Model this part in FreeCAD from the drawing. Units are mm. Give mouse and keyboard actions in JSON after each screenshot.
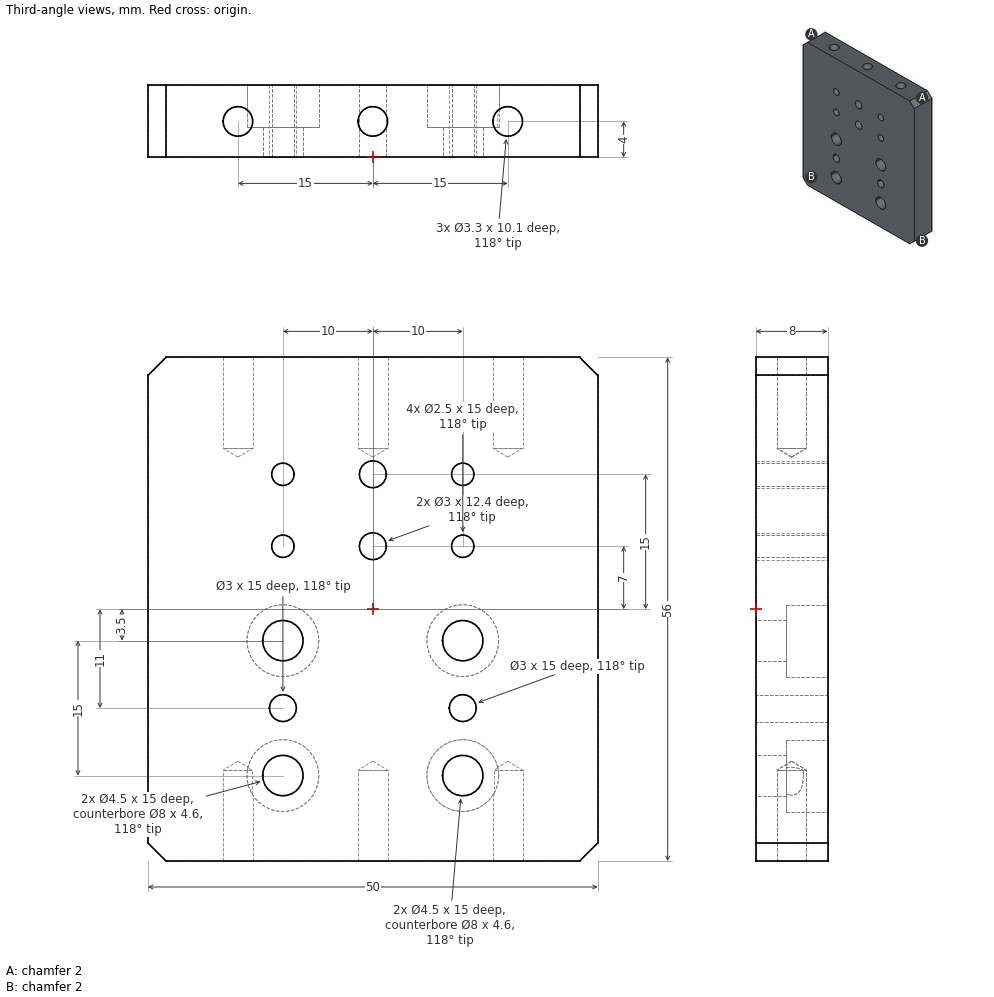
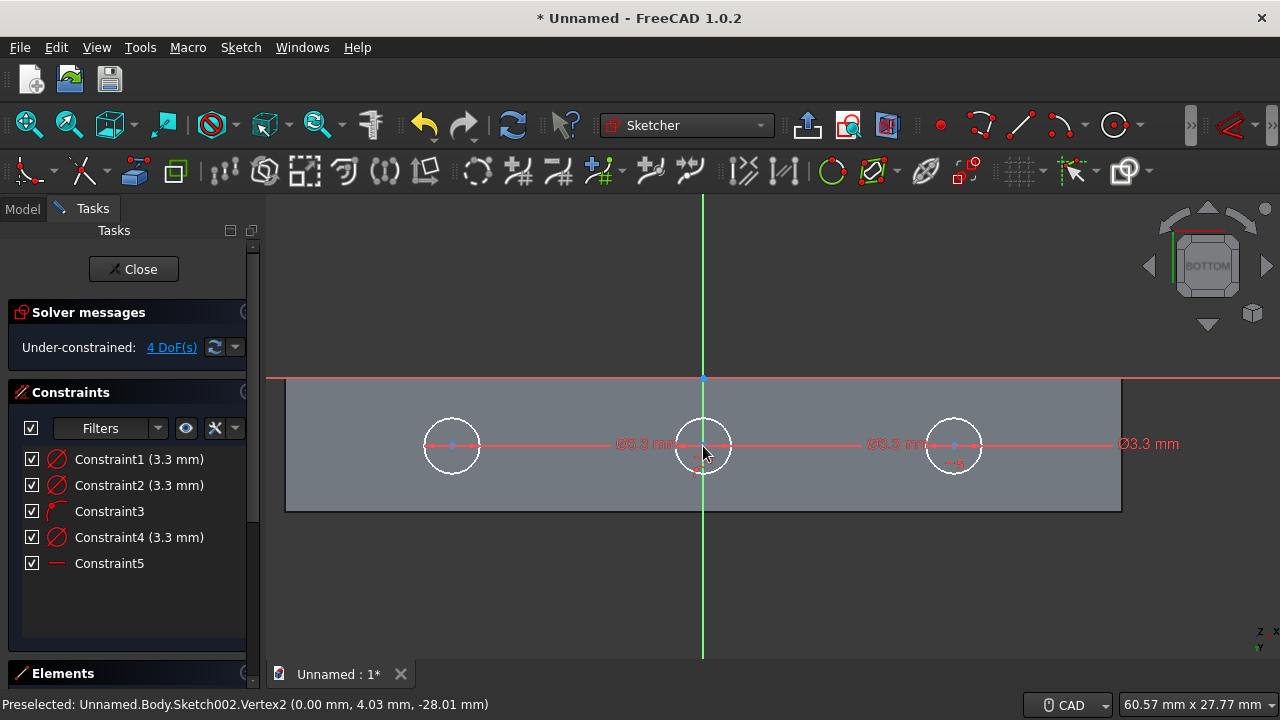
{"action": "left_click", "coordinate": [703, 446]}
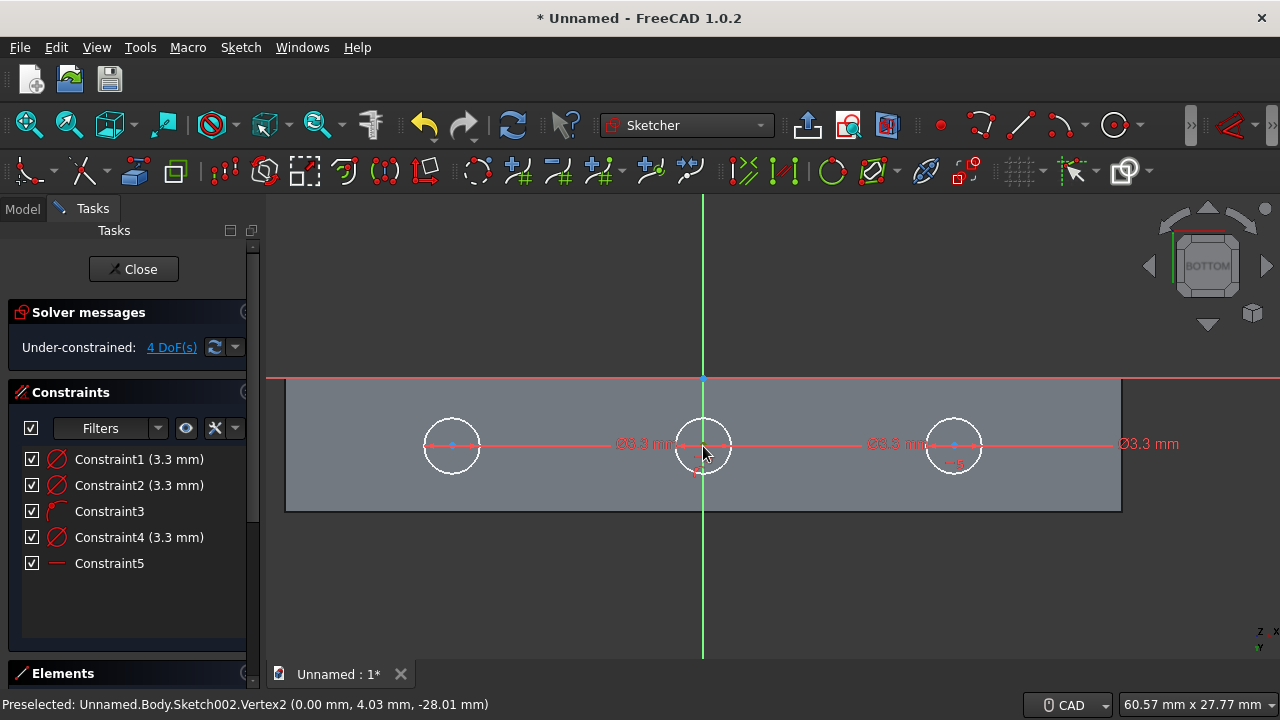
{"action": "left_click", "coordinate": [452, 446]}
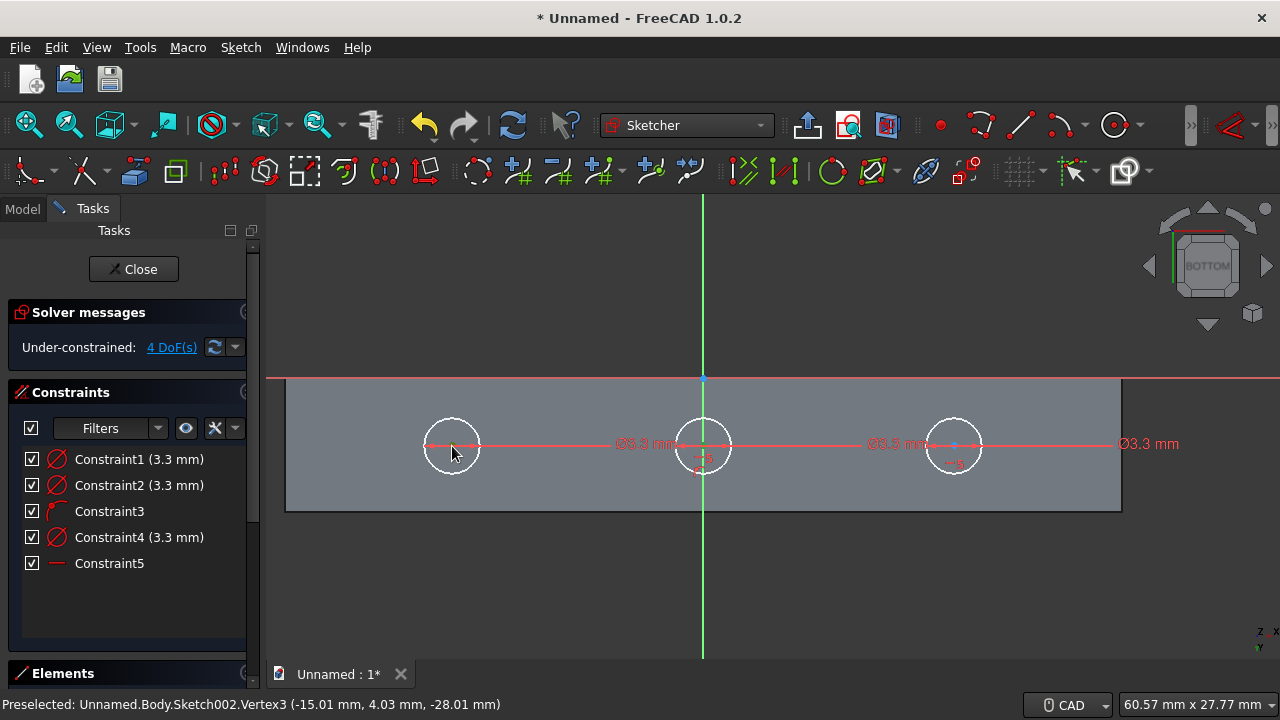
{"action": "key", "text": "h"}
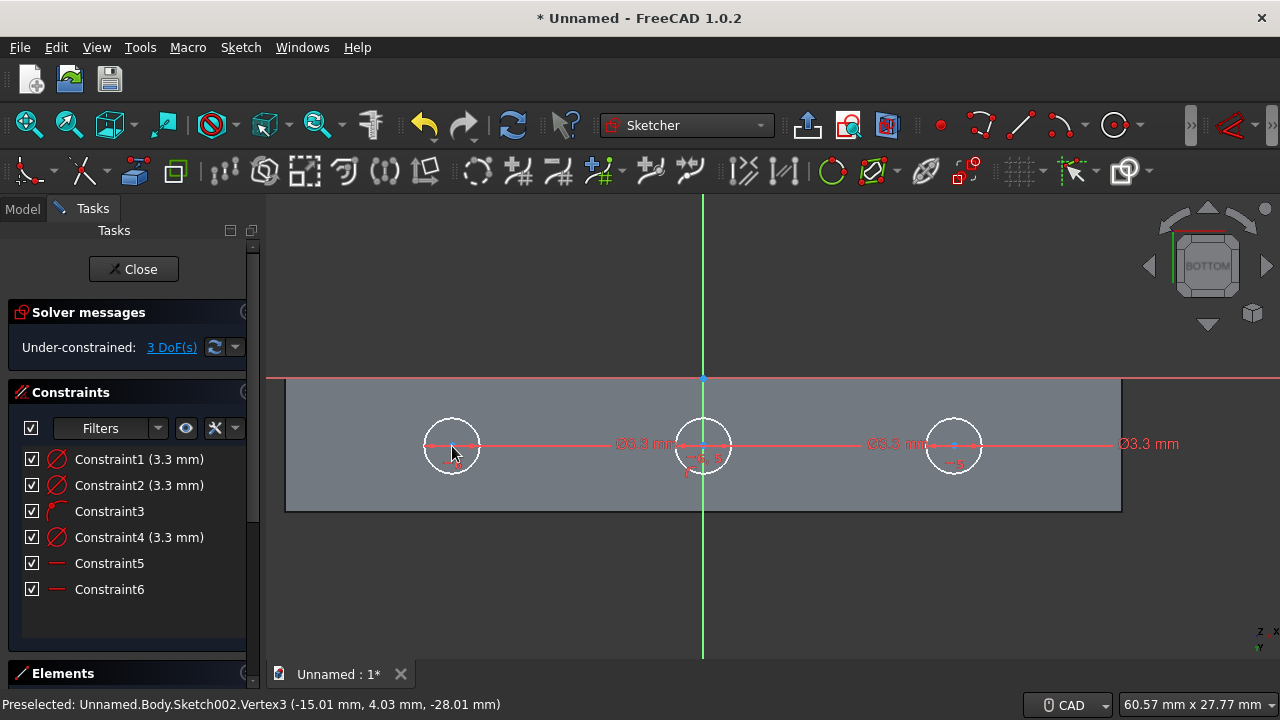
{"action": "left_click", "coordinate": [1230, 126]}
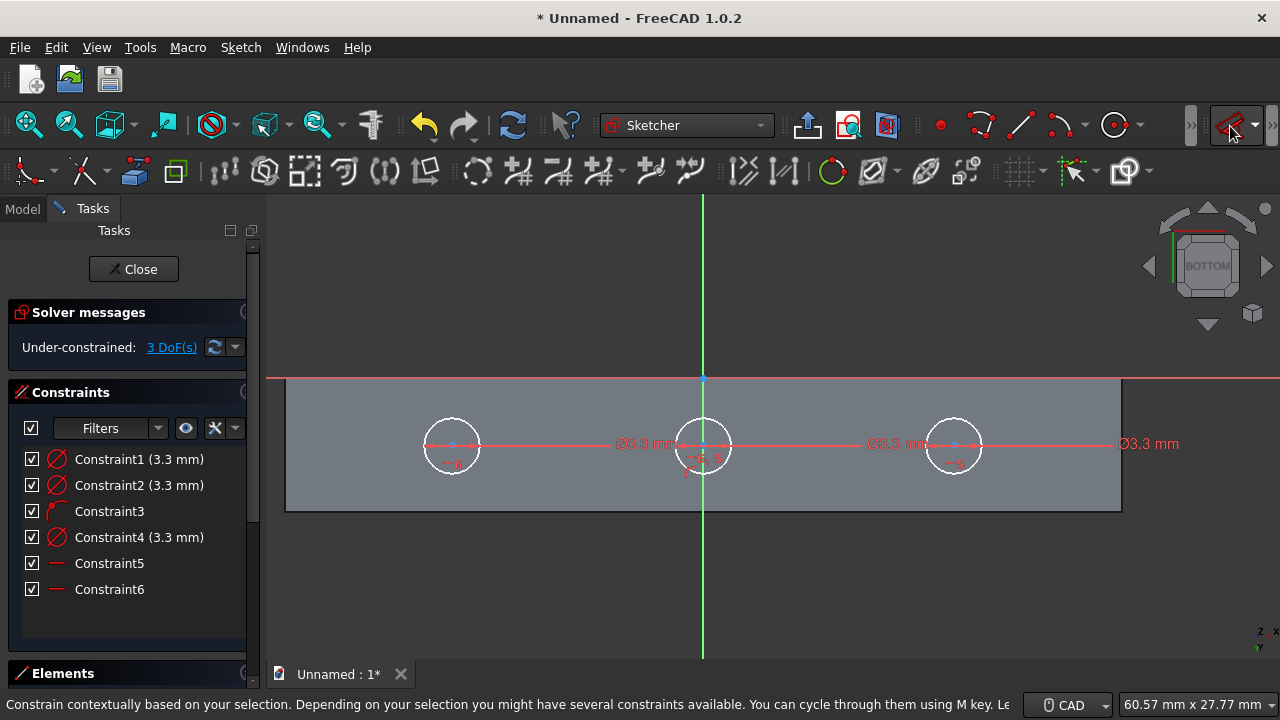
{"action": "left_click", "coordinate": [954, 446]}
{"action": "left_click", "coordinate": [988, 412]}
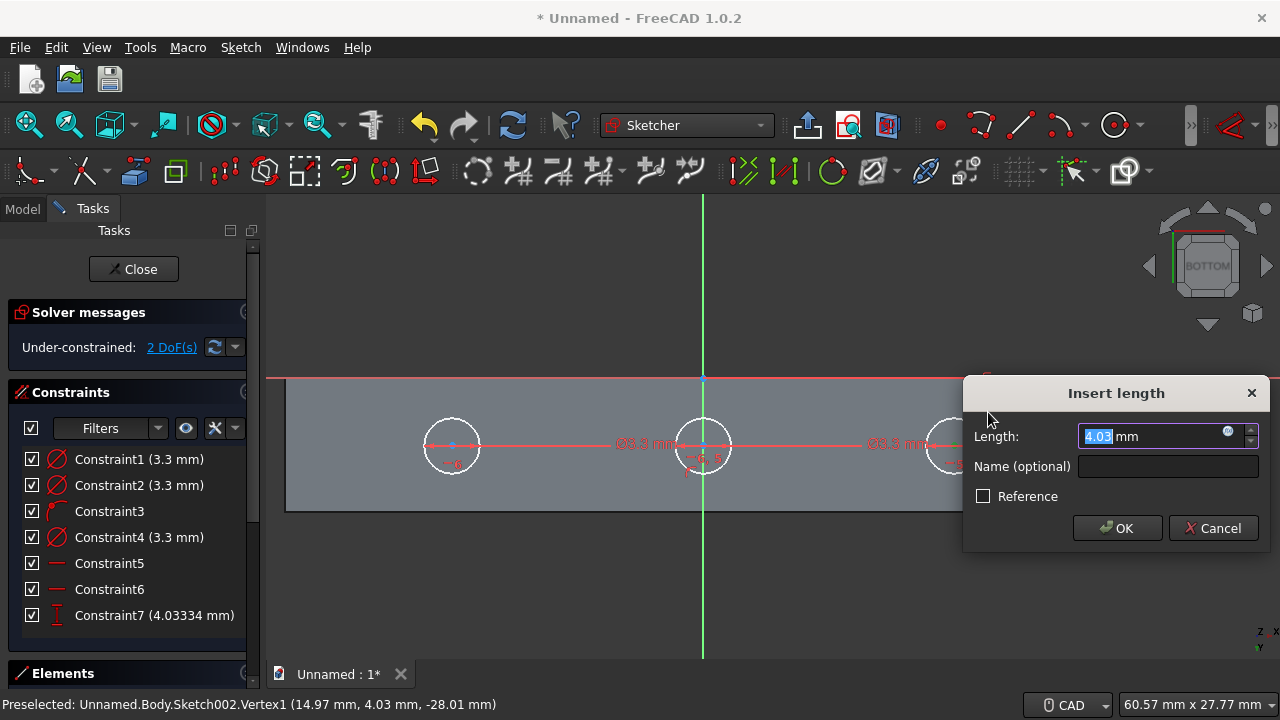
{"action": "type", "text": "4"}
{"action": "key", "text": "Return"}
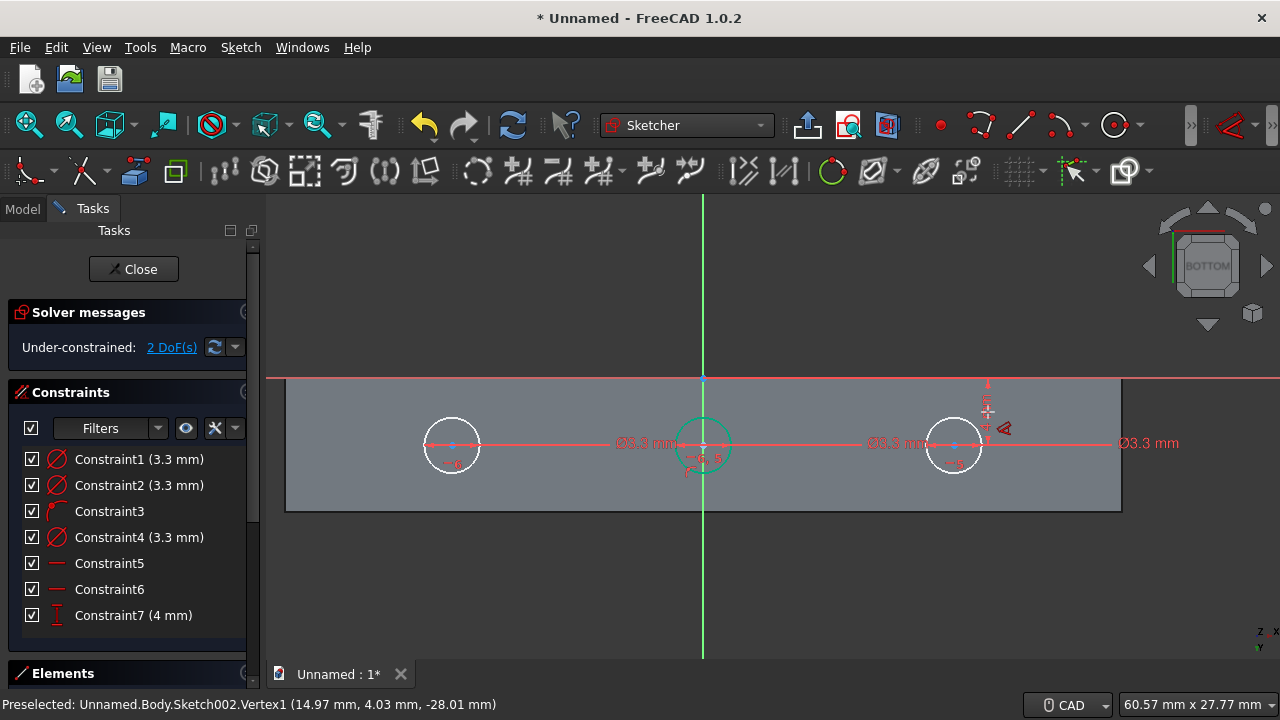
{"action": "left_click", "coordinate": [954, 445]}
{"action": "left_click", "coordinate": [829, 344]}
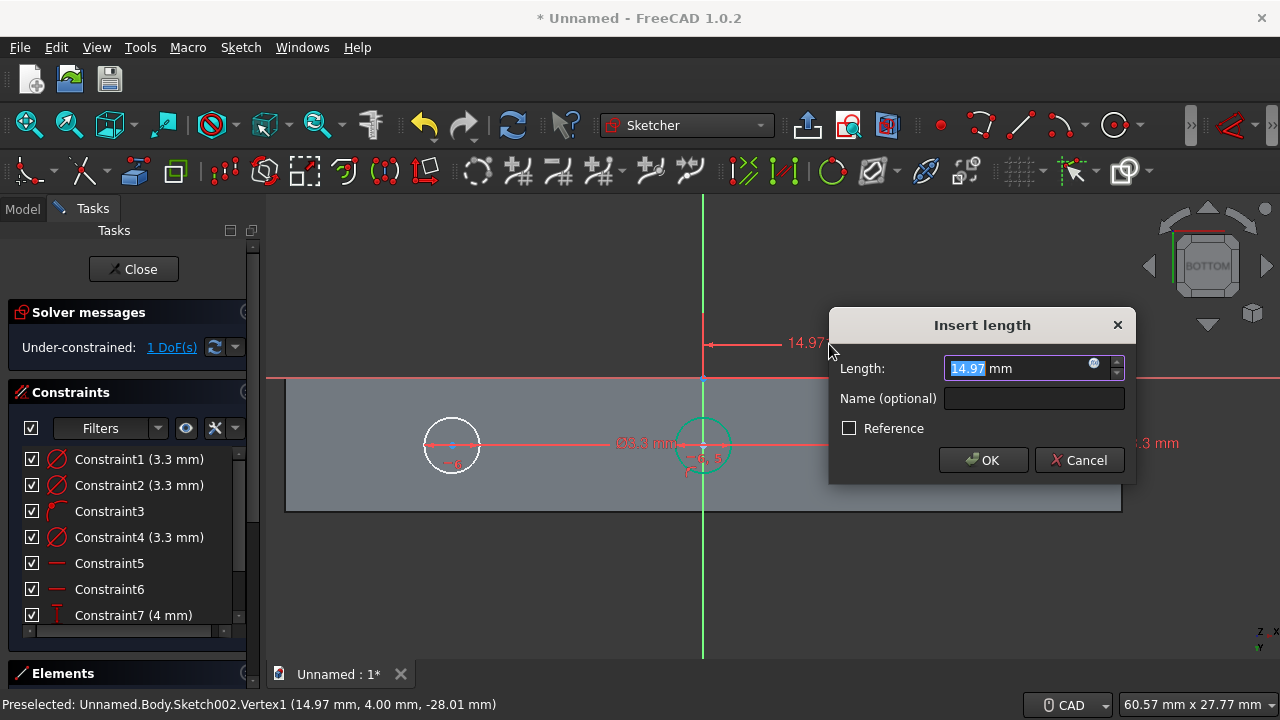
{"action": "type", "text": "15"}
{"action": "key", "text": "Return"}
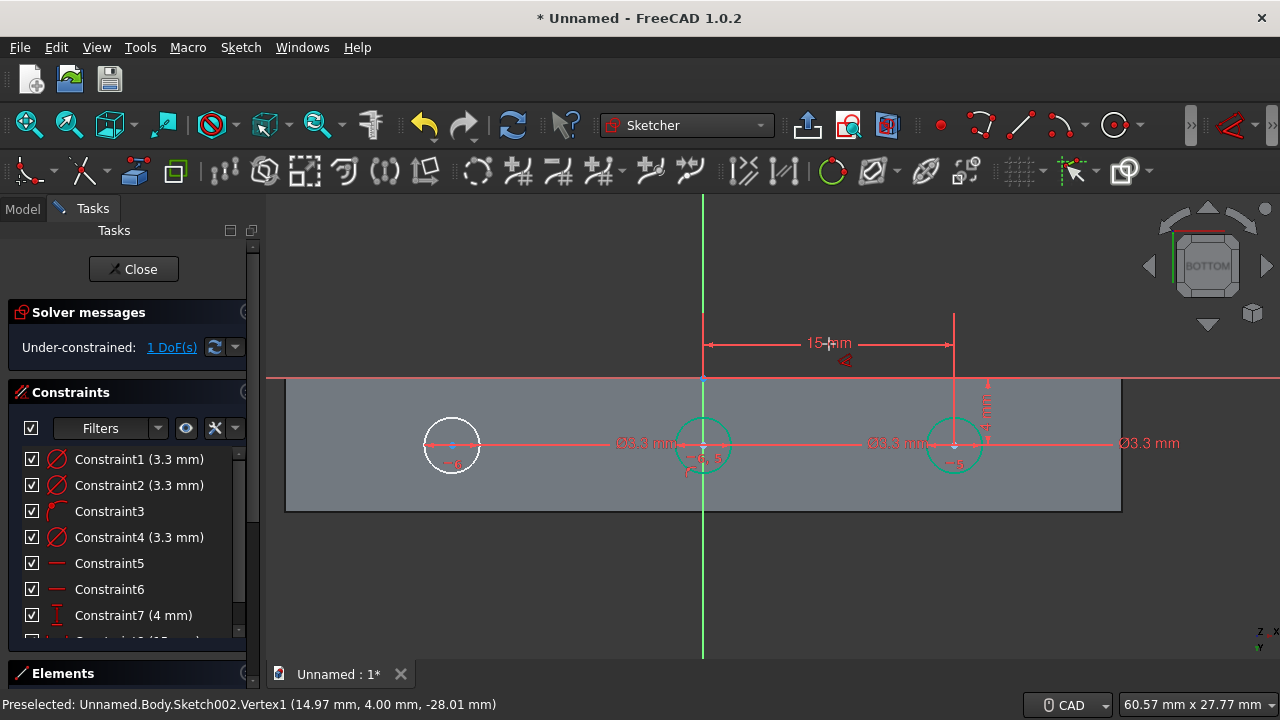
{"action": "left_click", "coordinate": [452, 445]}
{"action": "left_click", "coordinate": [578, 344]}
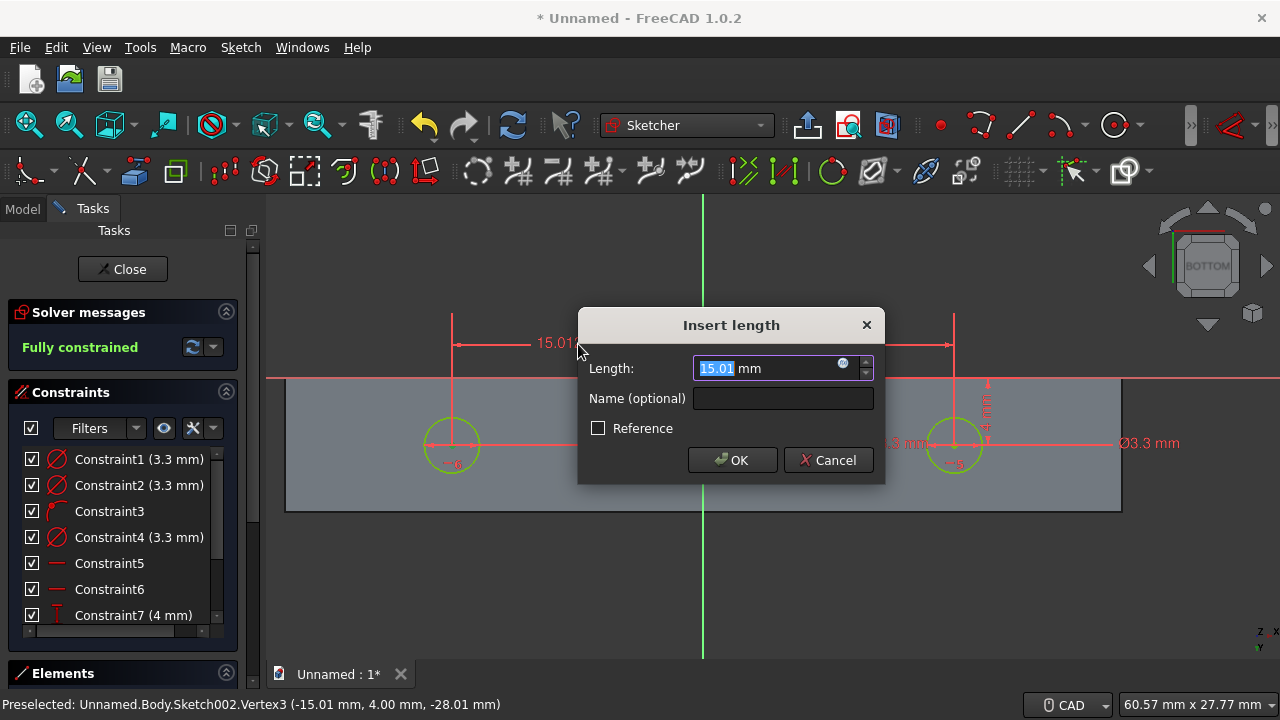
{"action": "type", "text": "15"}
{"action": "key", "text": "Return"}
{"action": "key", "text": "Escape"}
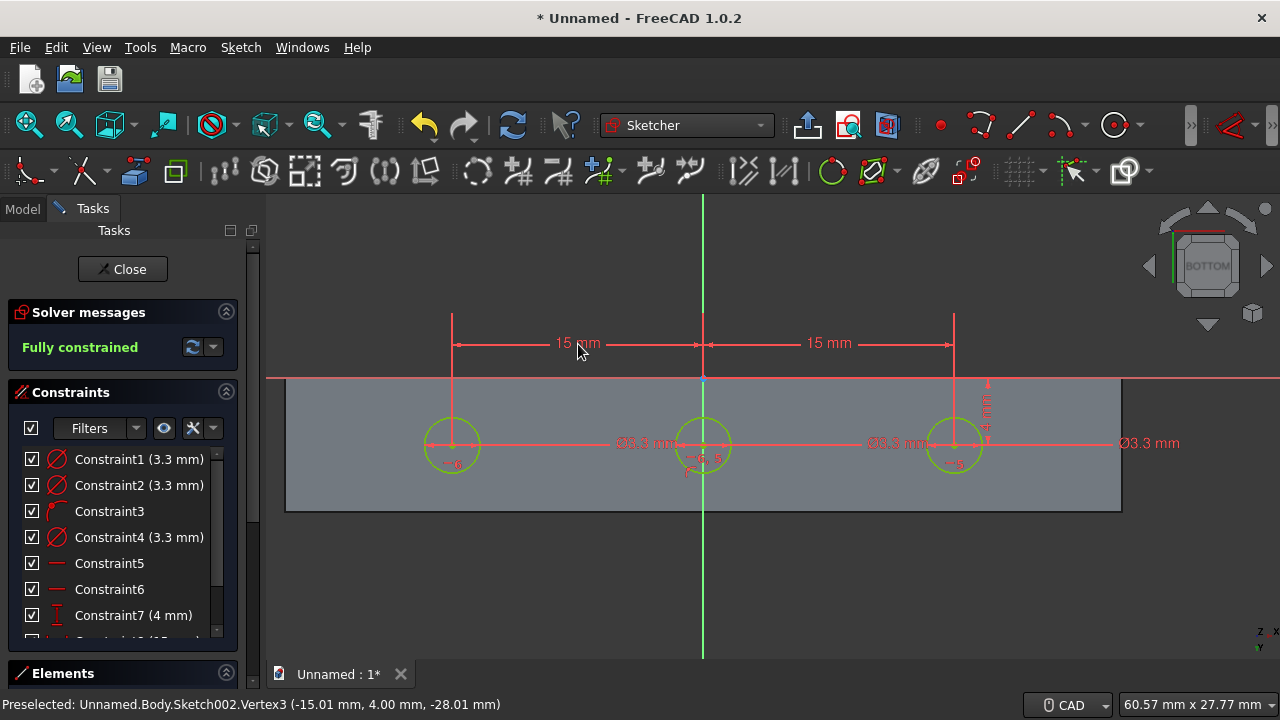
{"action": "left_click", "coordinate": [123, 269]}